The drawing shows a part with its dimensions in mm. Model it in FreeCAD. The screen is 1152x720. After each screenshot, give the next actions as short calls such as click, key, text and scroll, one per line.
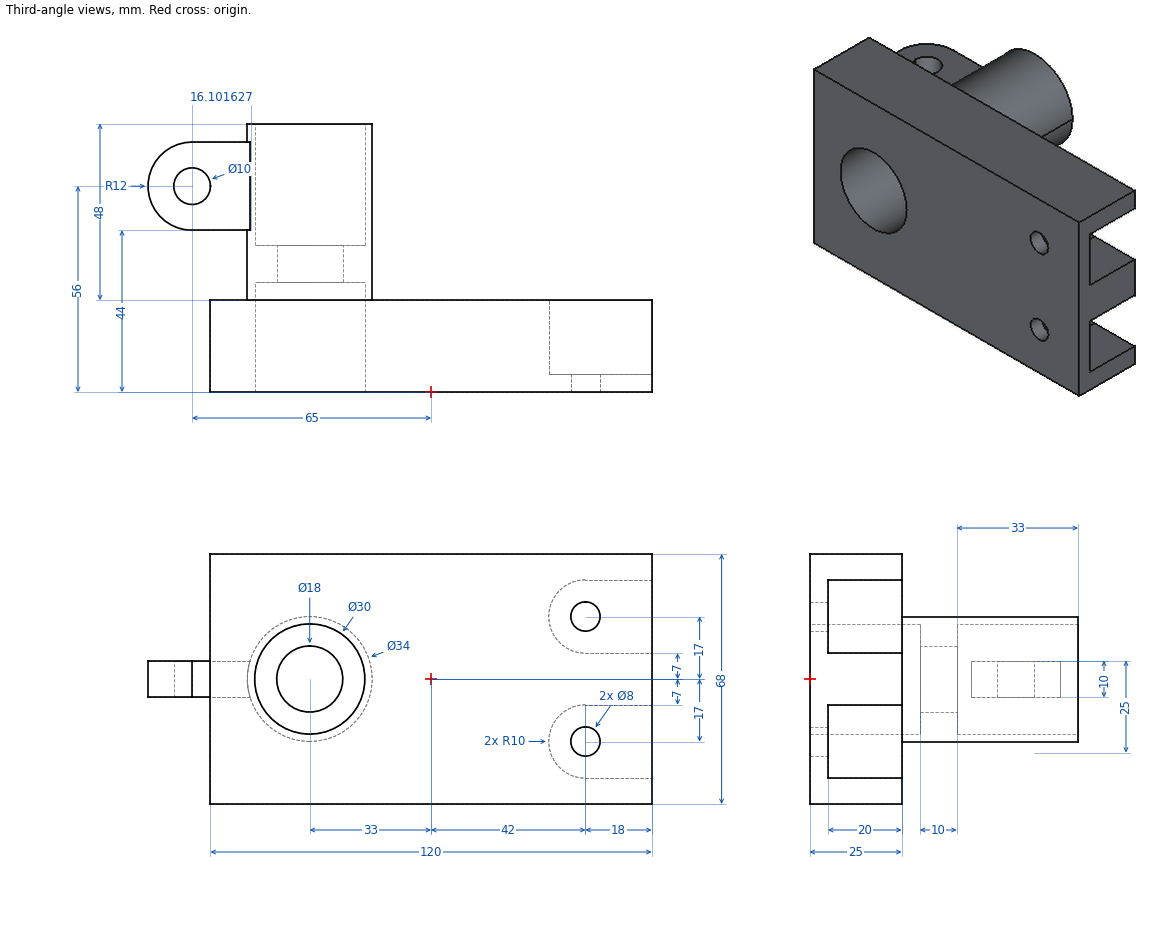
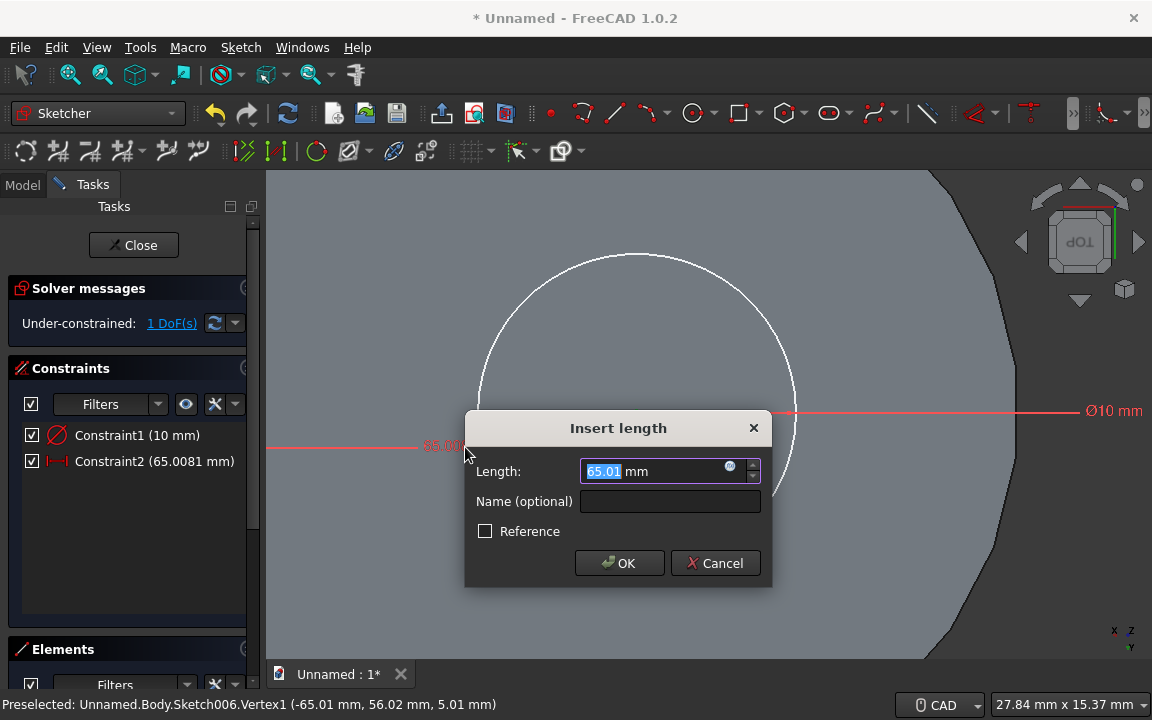
text(65)
key(Return)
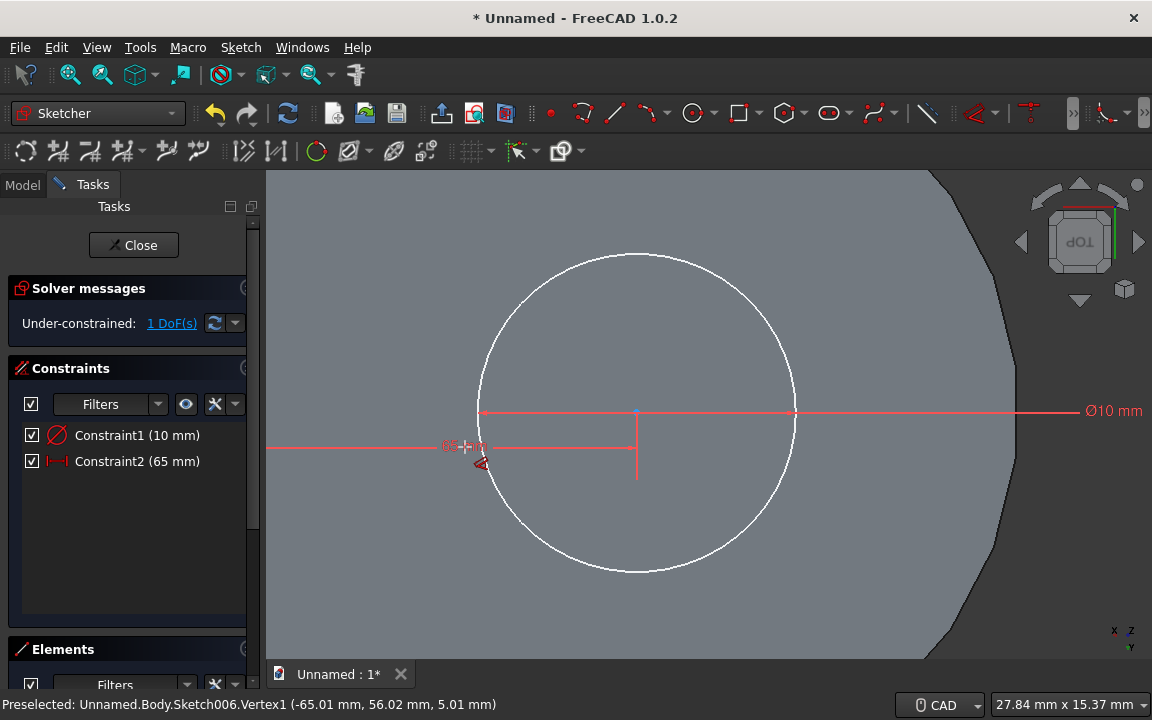
click(637, 413)
click(671, 305)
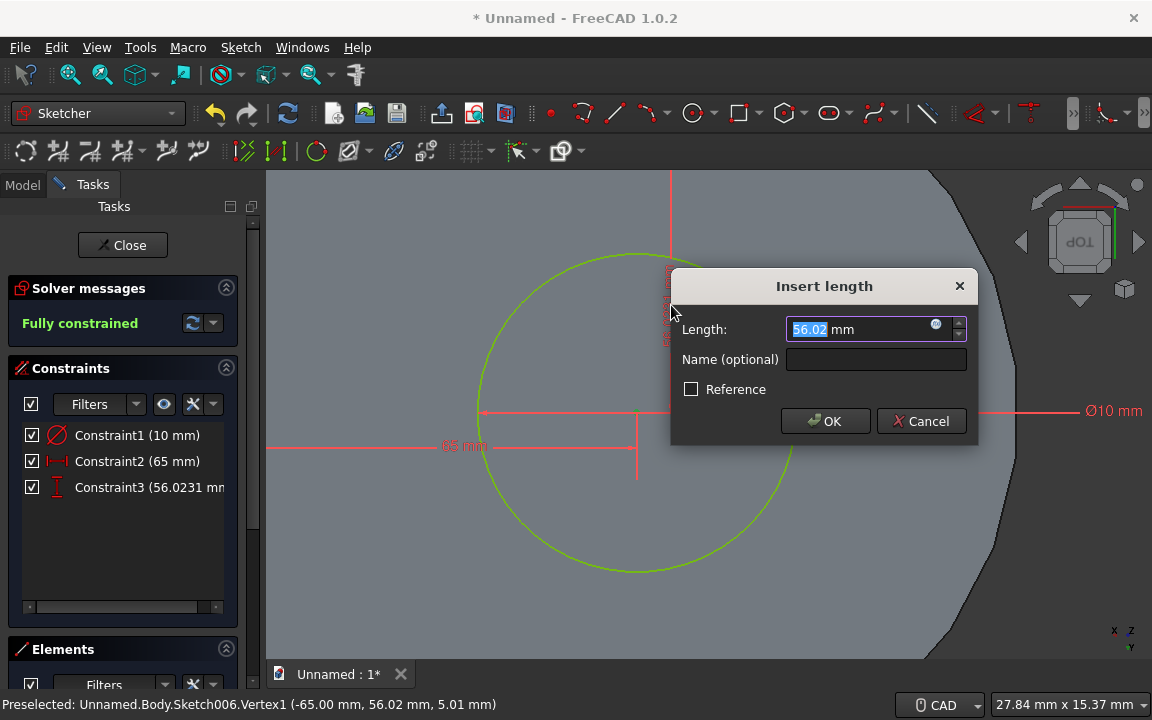
text(56)
key(Return)
key(Escape)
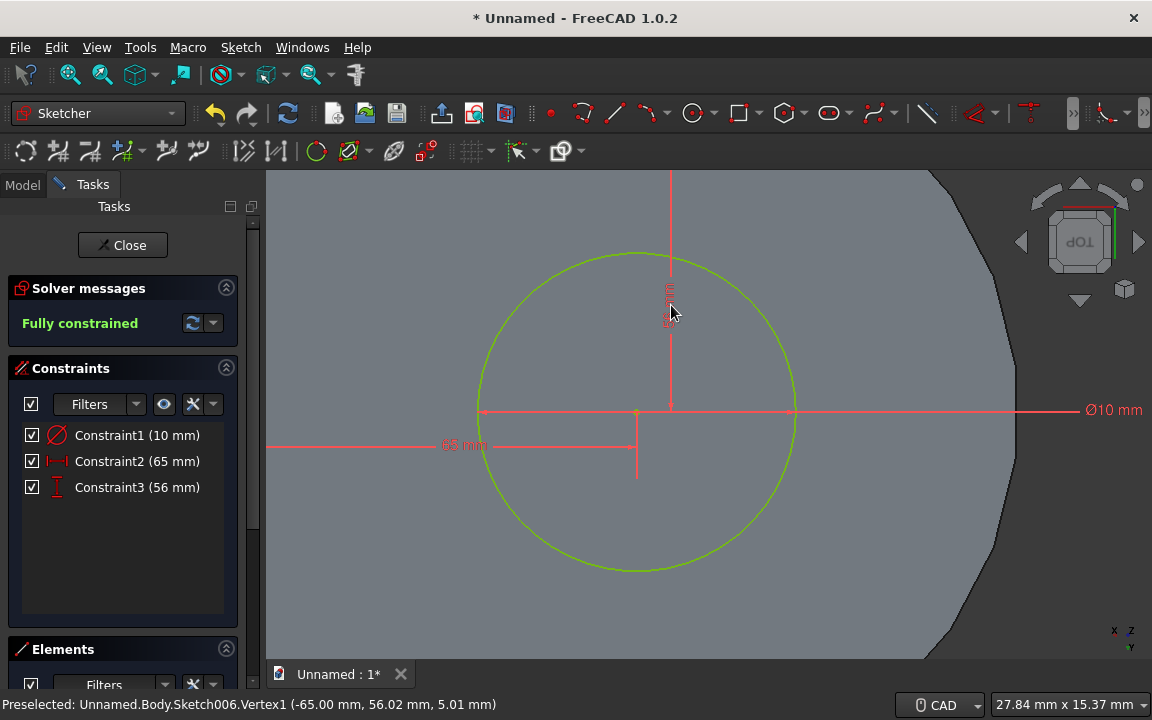
click(123, 245)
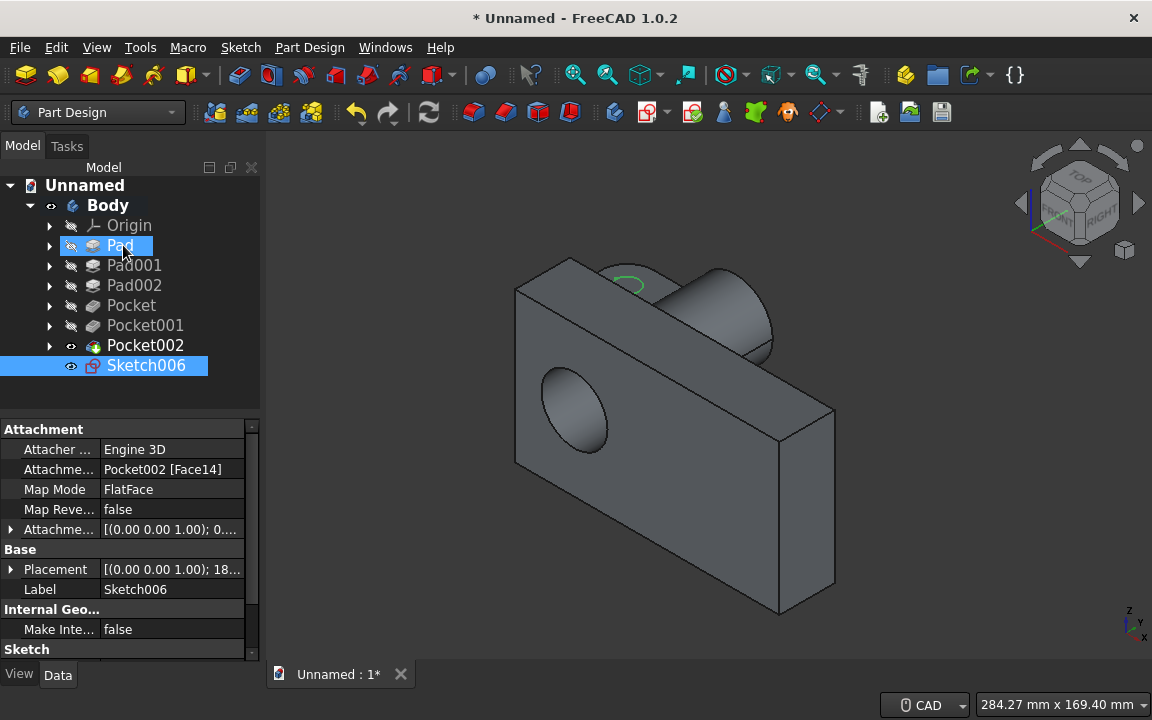
click(240, 76)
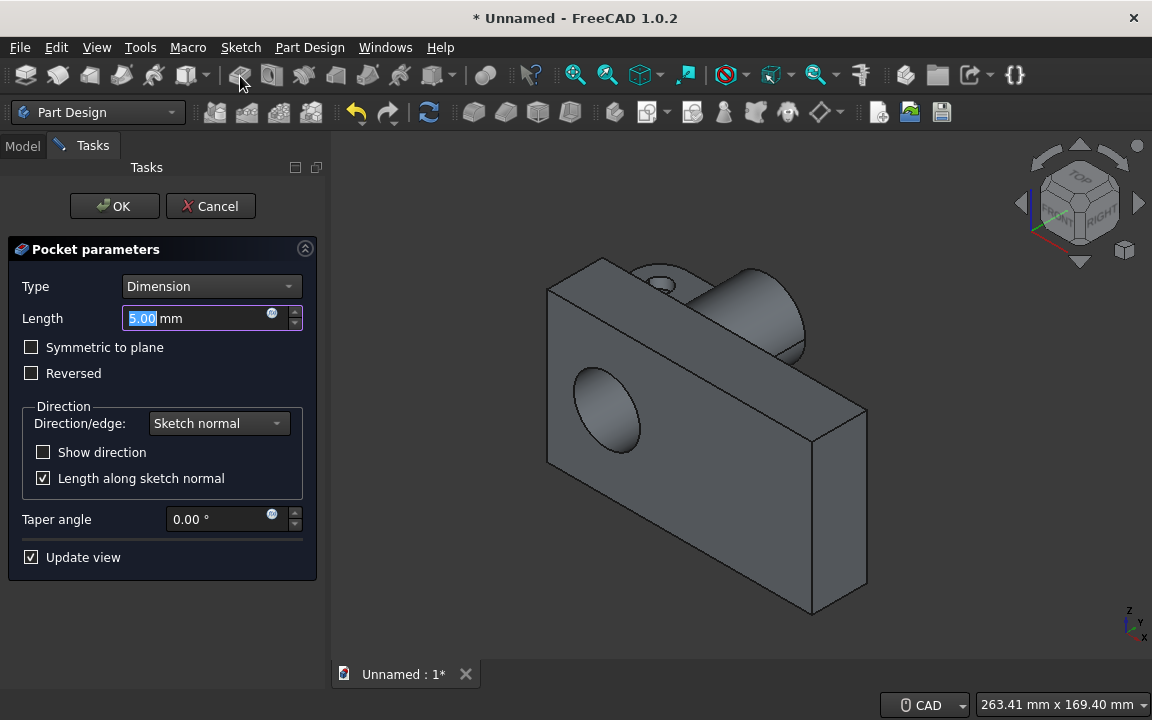
text(25)
key(Tab)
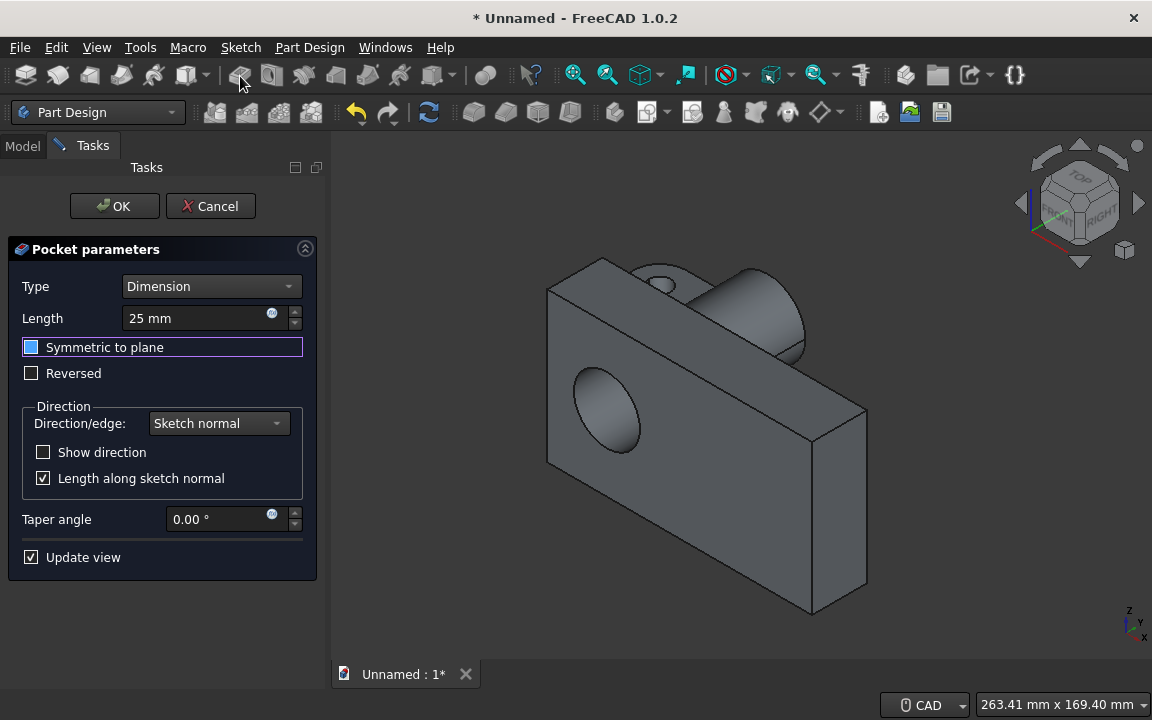
click(115, 206)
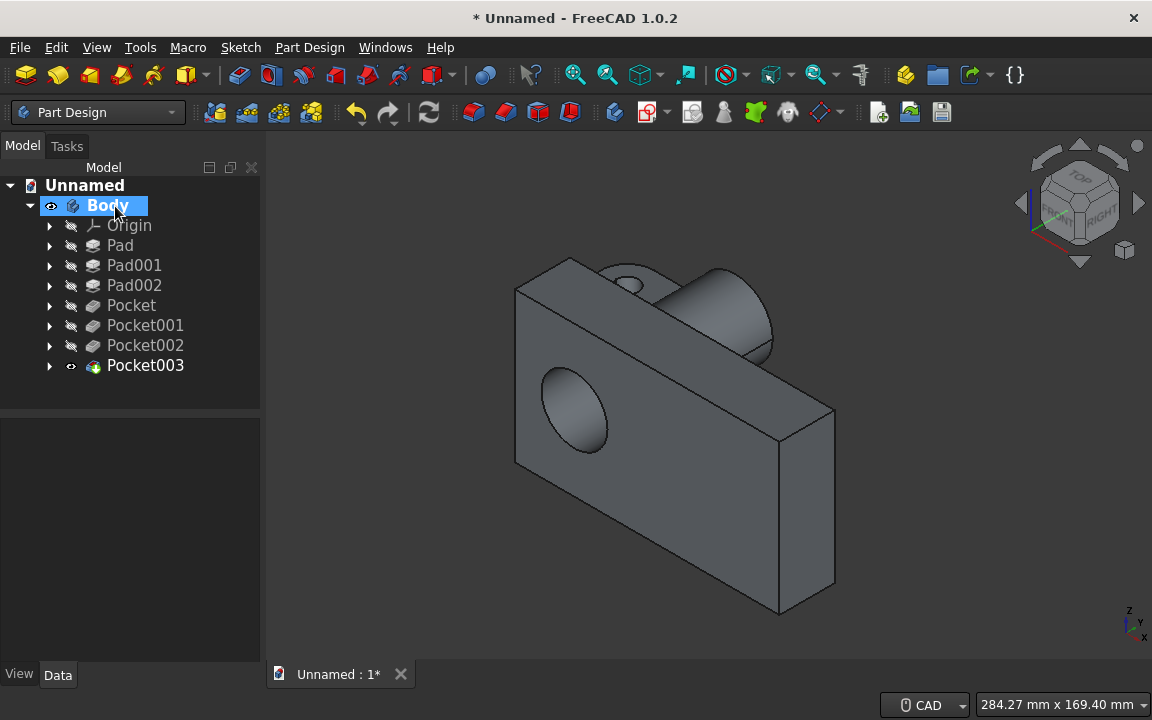
key(4)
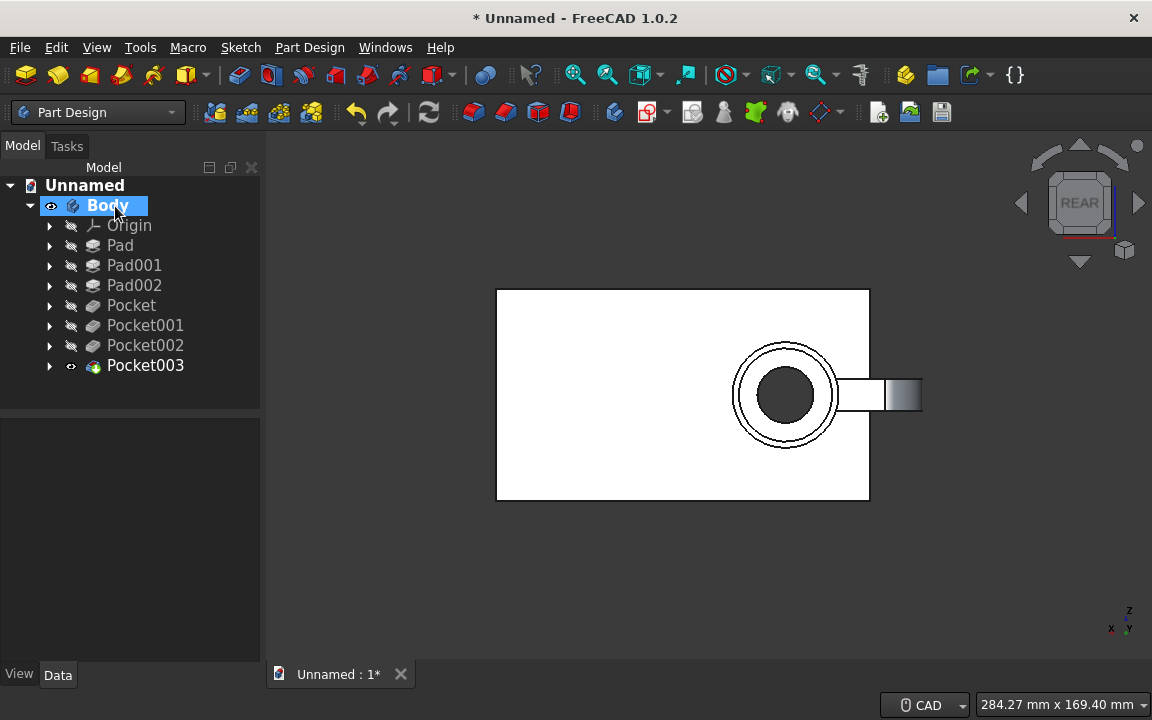
click(629, 394)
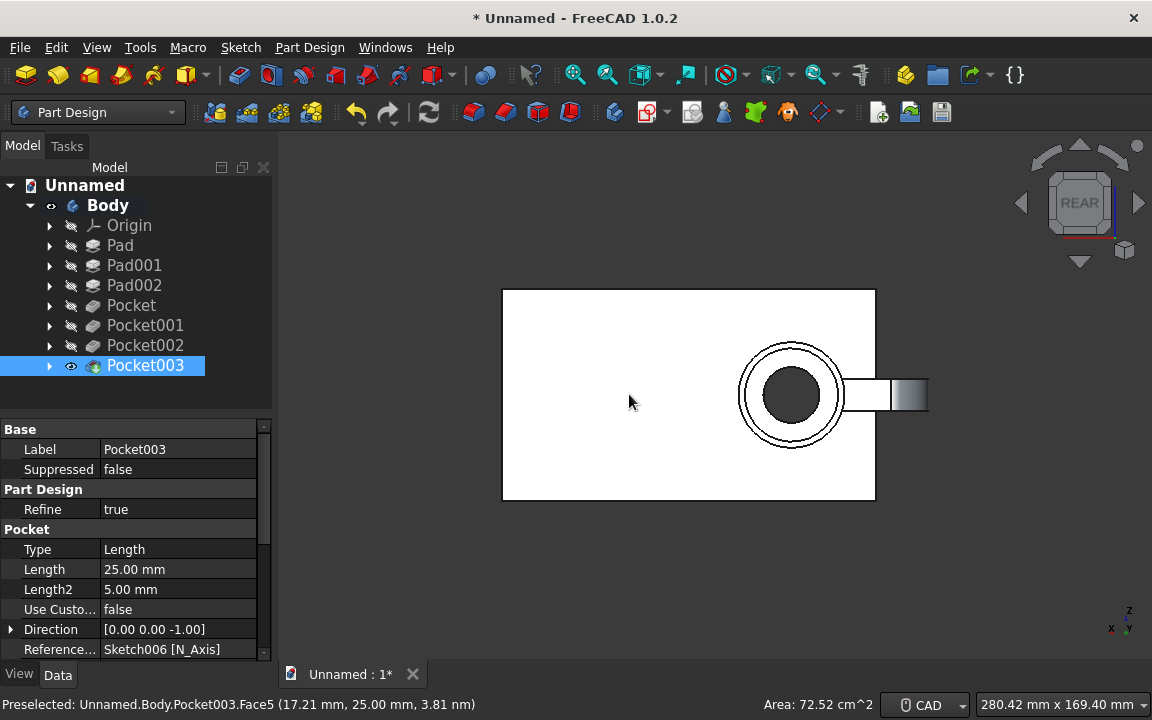
click(648, 112)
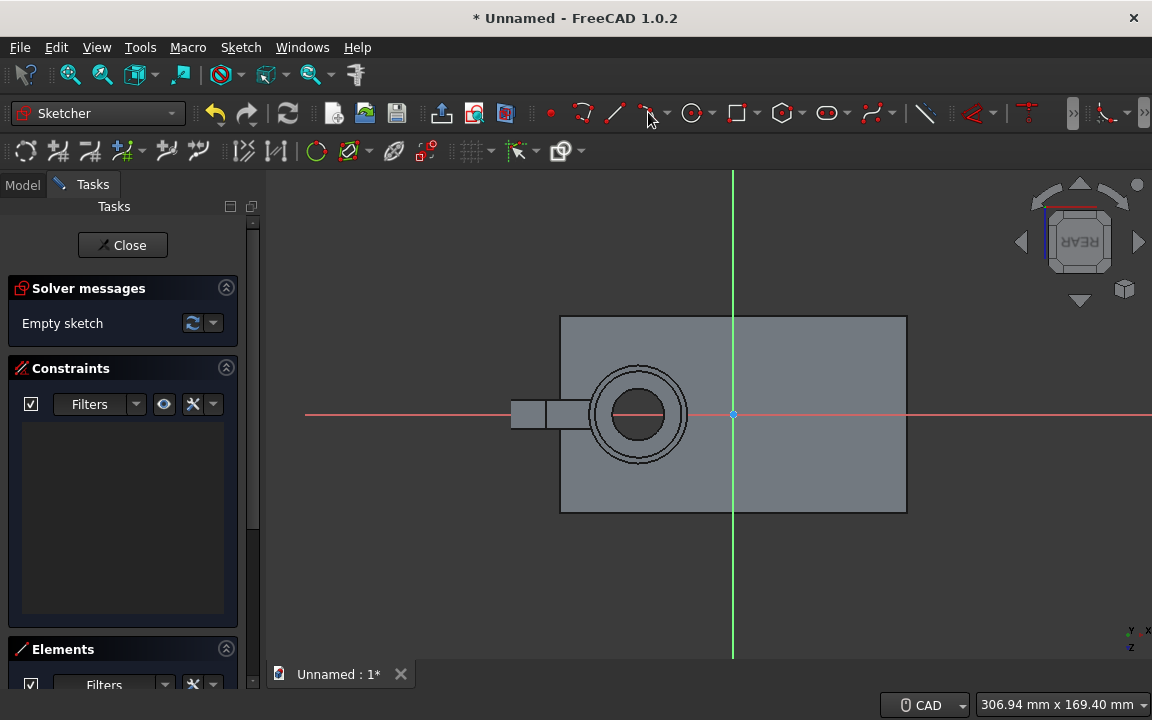
scroll(987, 415, up, 3)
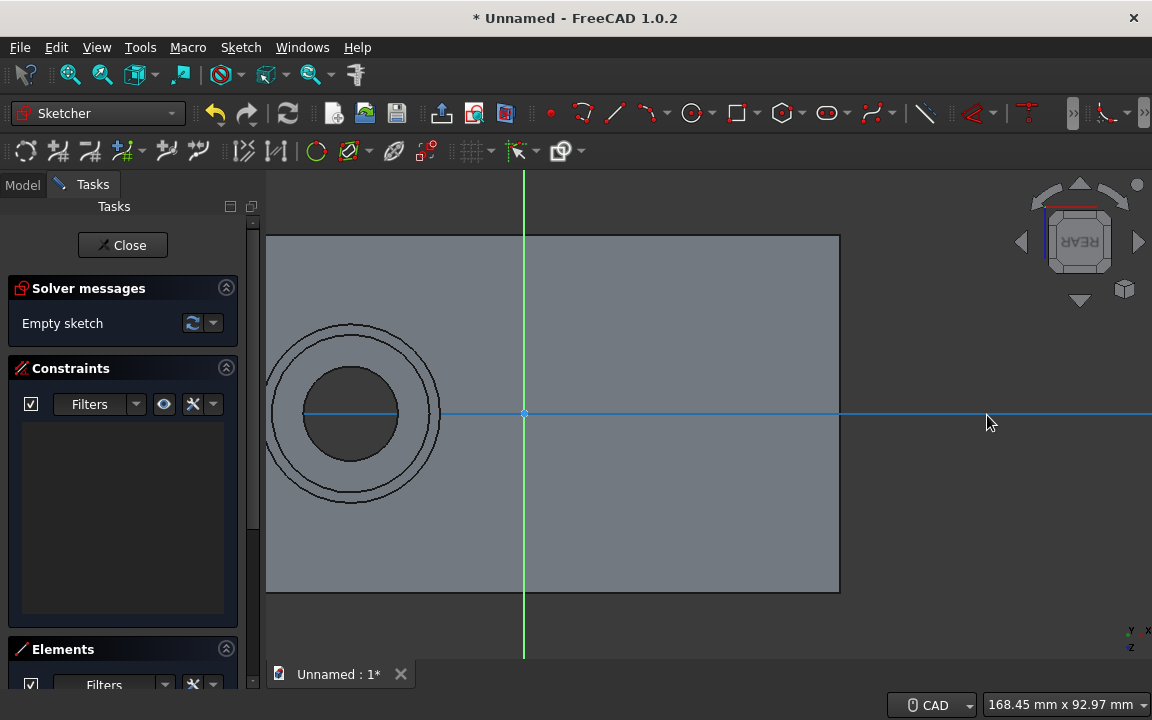
click(584, 114)